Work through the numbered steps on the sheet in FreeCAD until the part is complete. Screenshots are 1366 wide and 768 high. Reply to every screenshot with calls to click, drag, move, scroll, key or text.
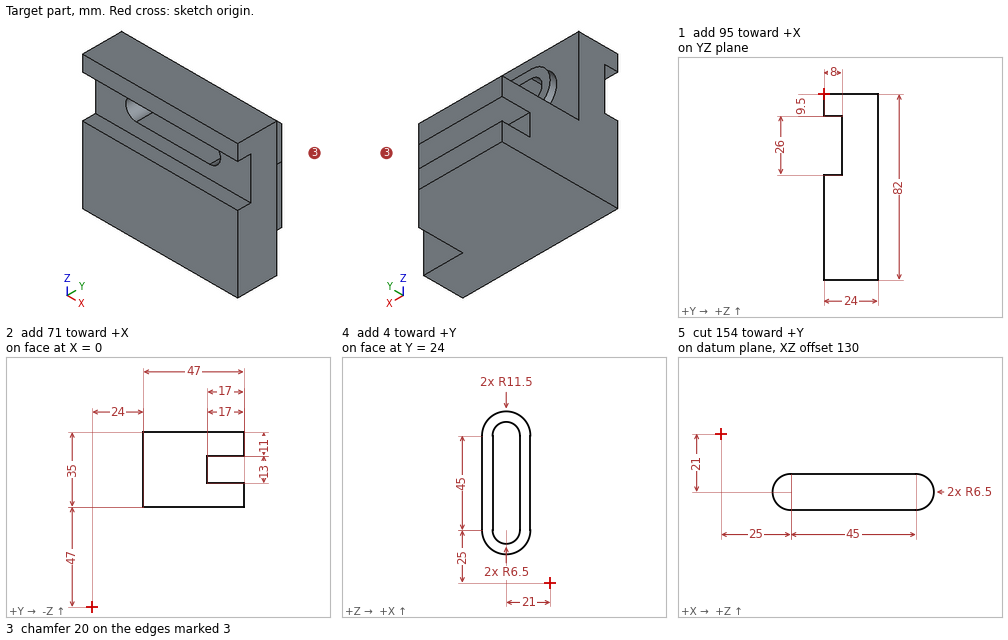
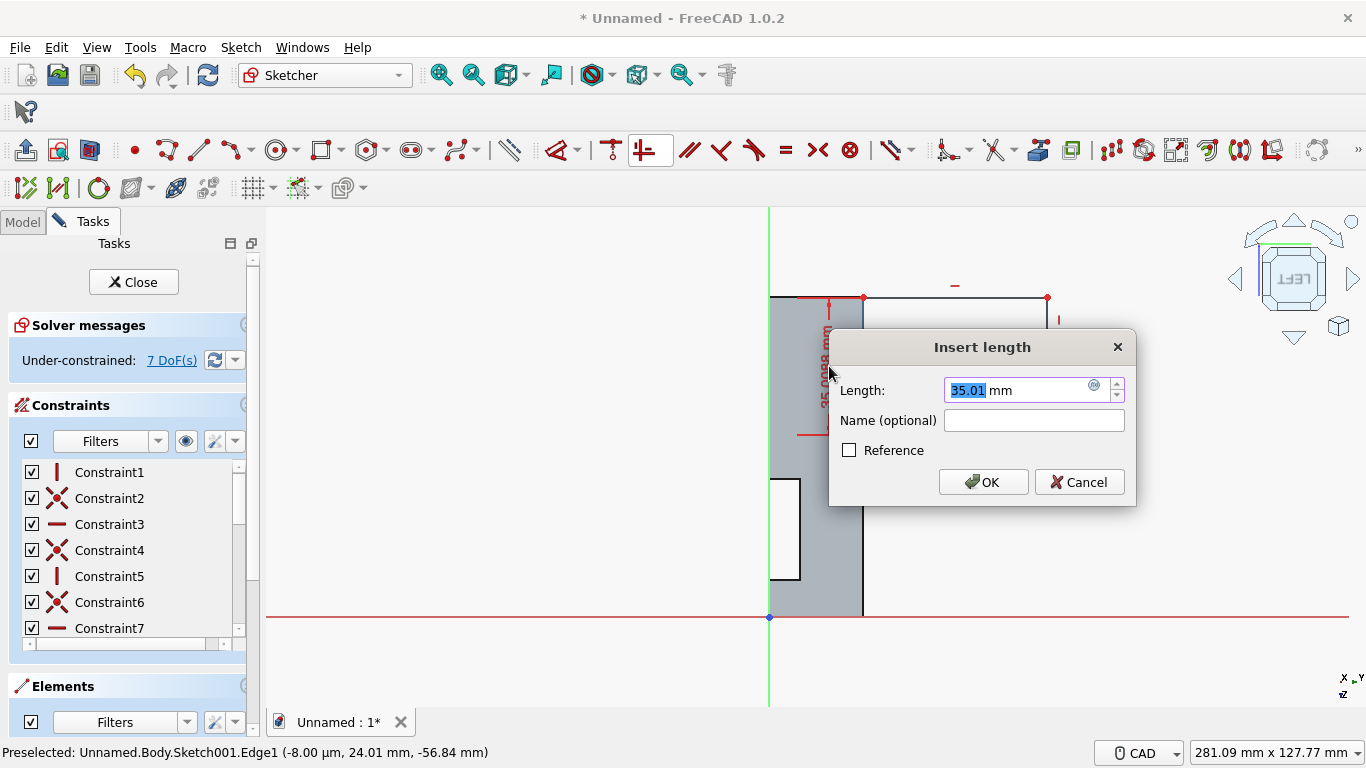
text(35)
key(Return)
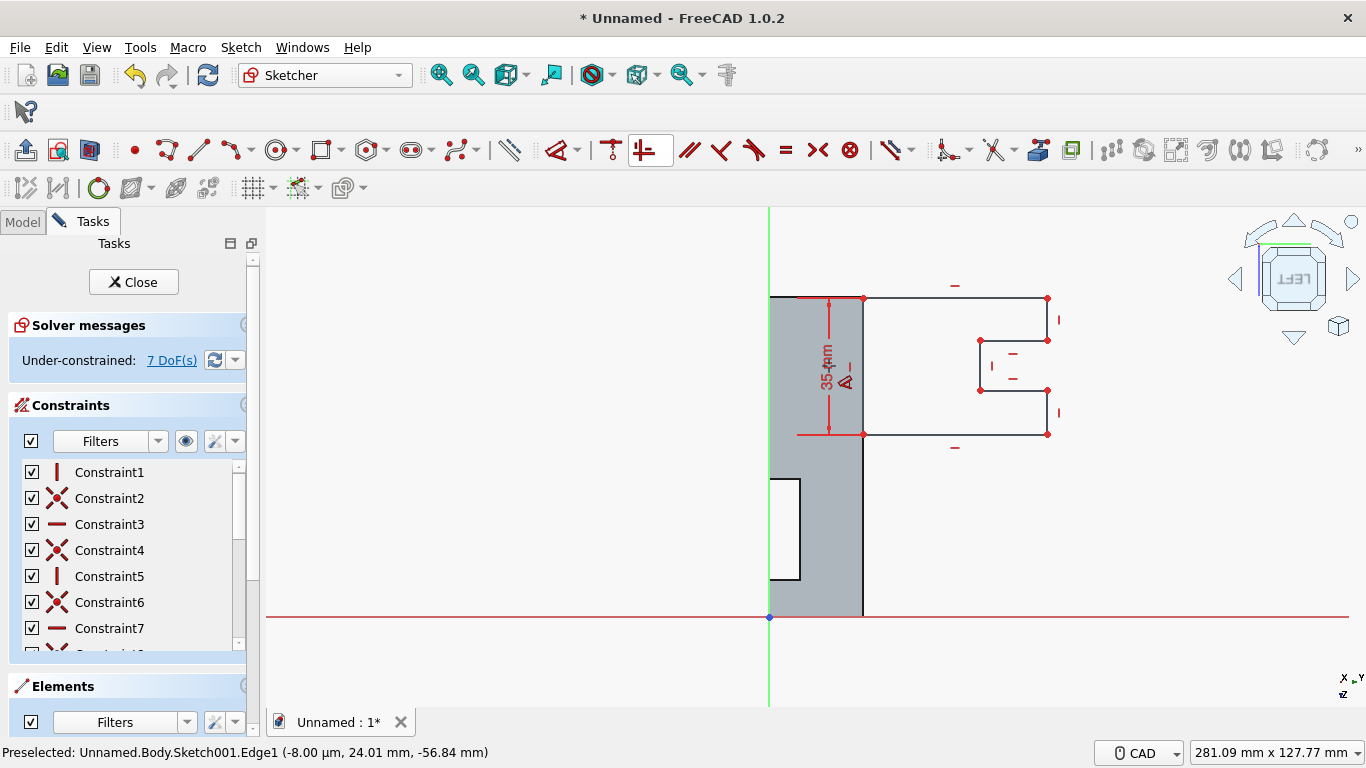
click(918, 298)
click(955, 264)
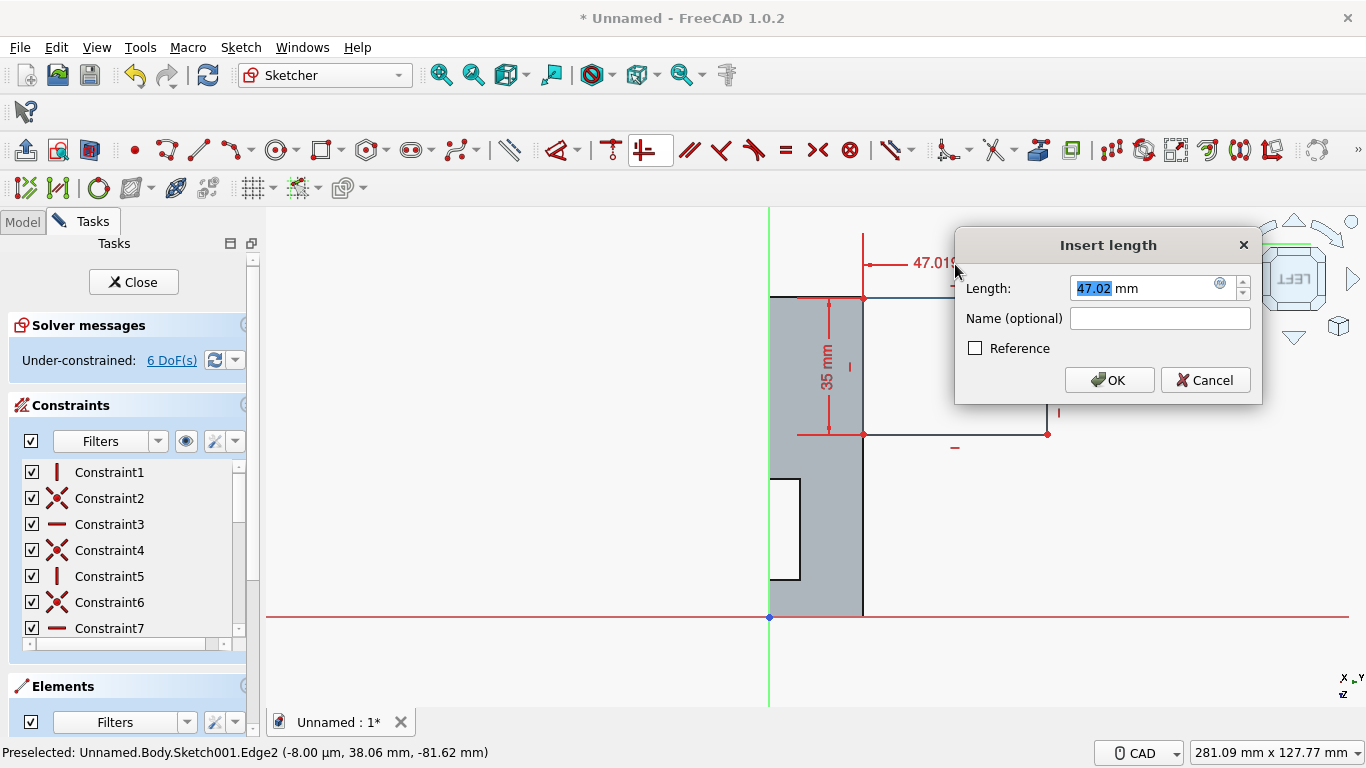
text(47)
key(Return)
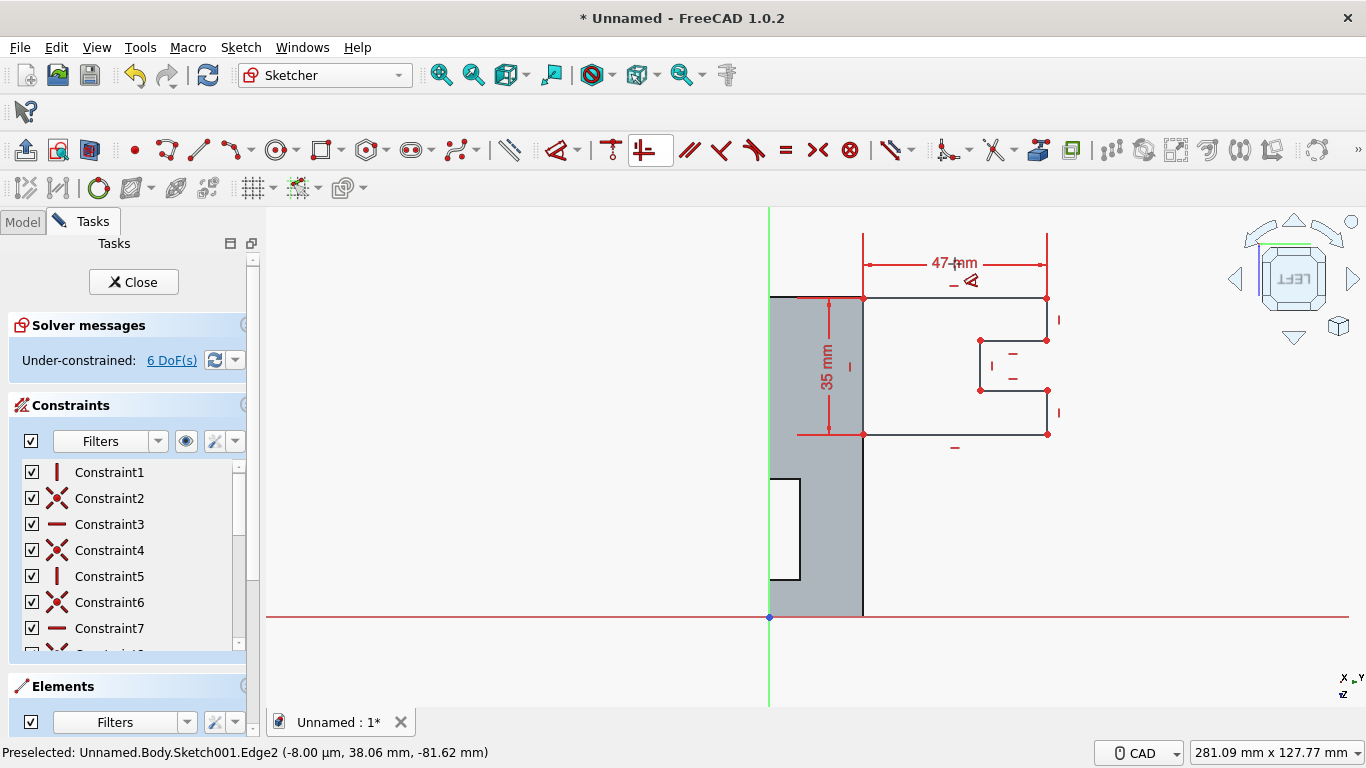
click(1047, 311)
click(1081, 320)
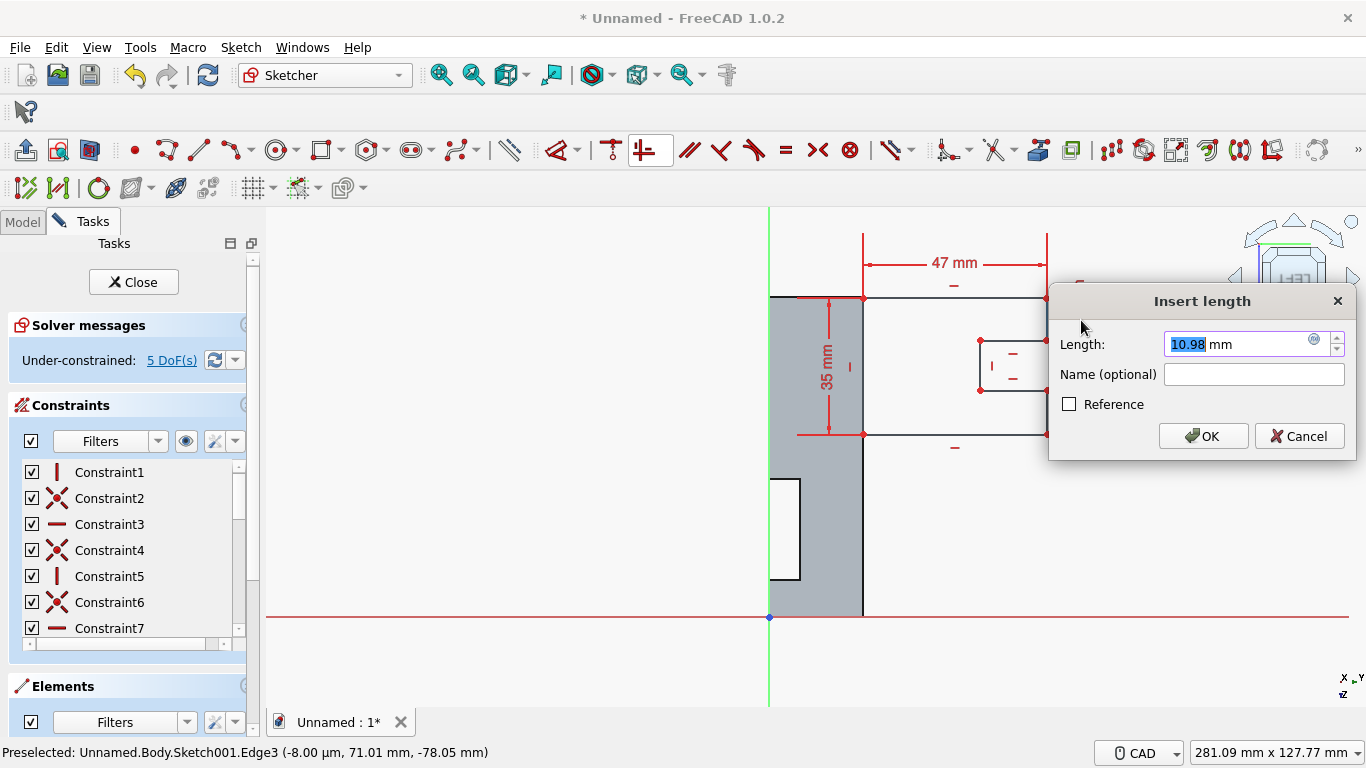
text(11)
key(Return)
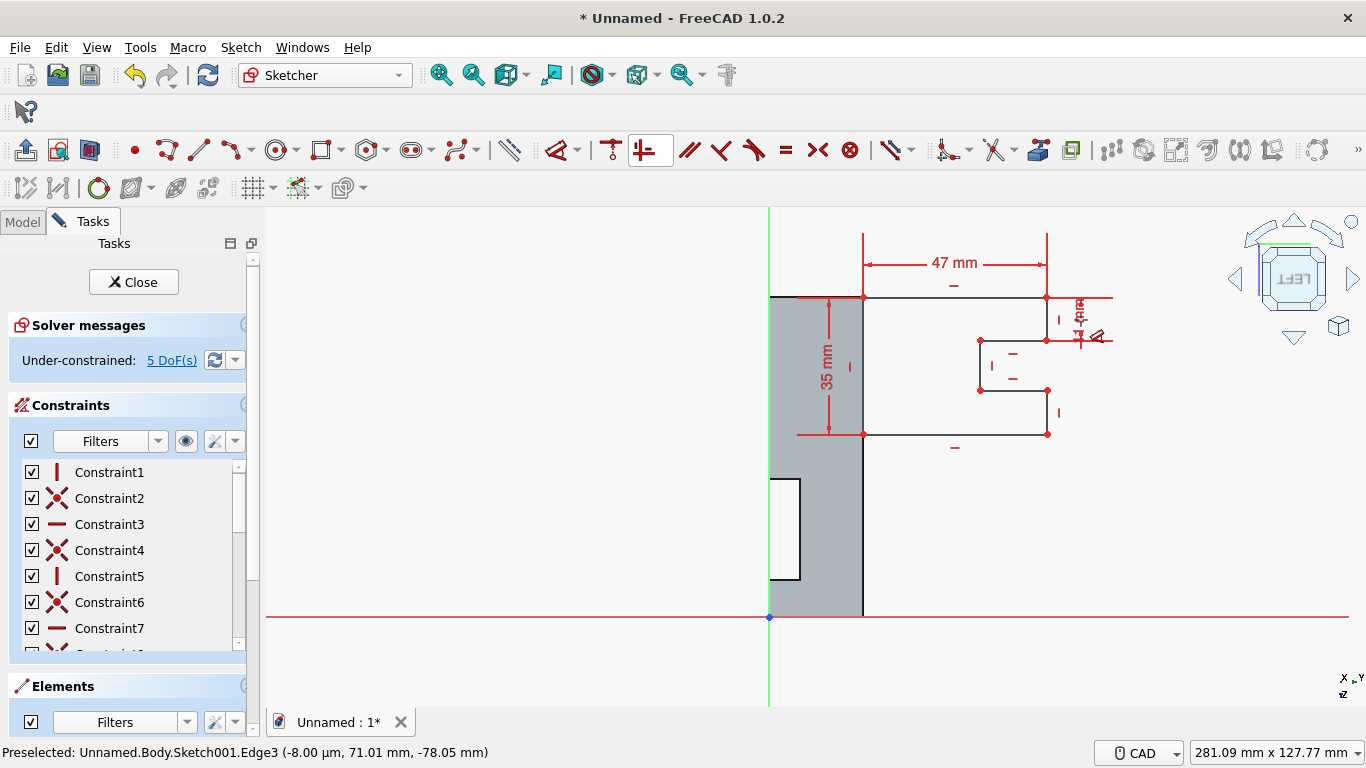
click(1027, 341)
click(1013, 375)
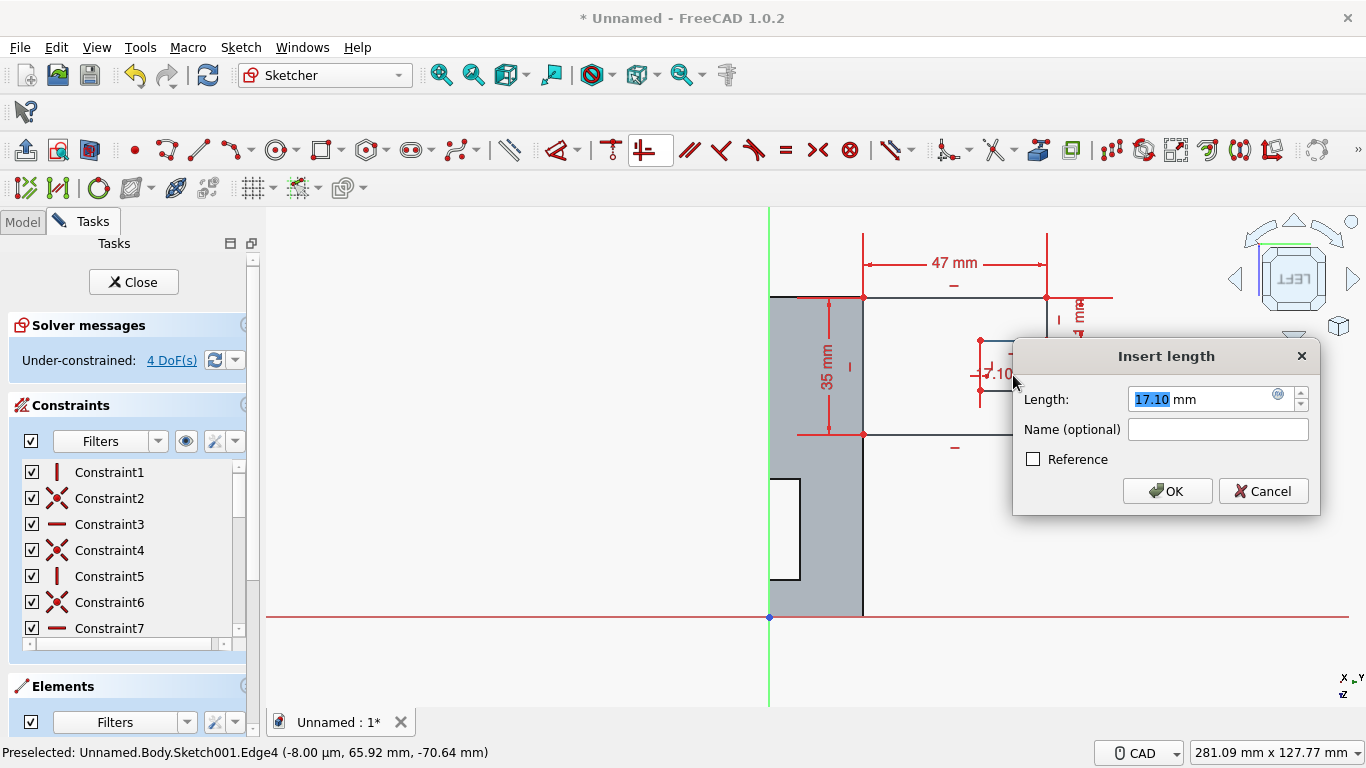
text(17)
key(Return)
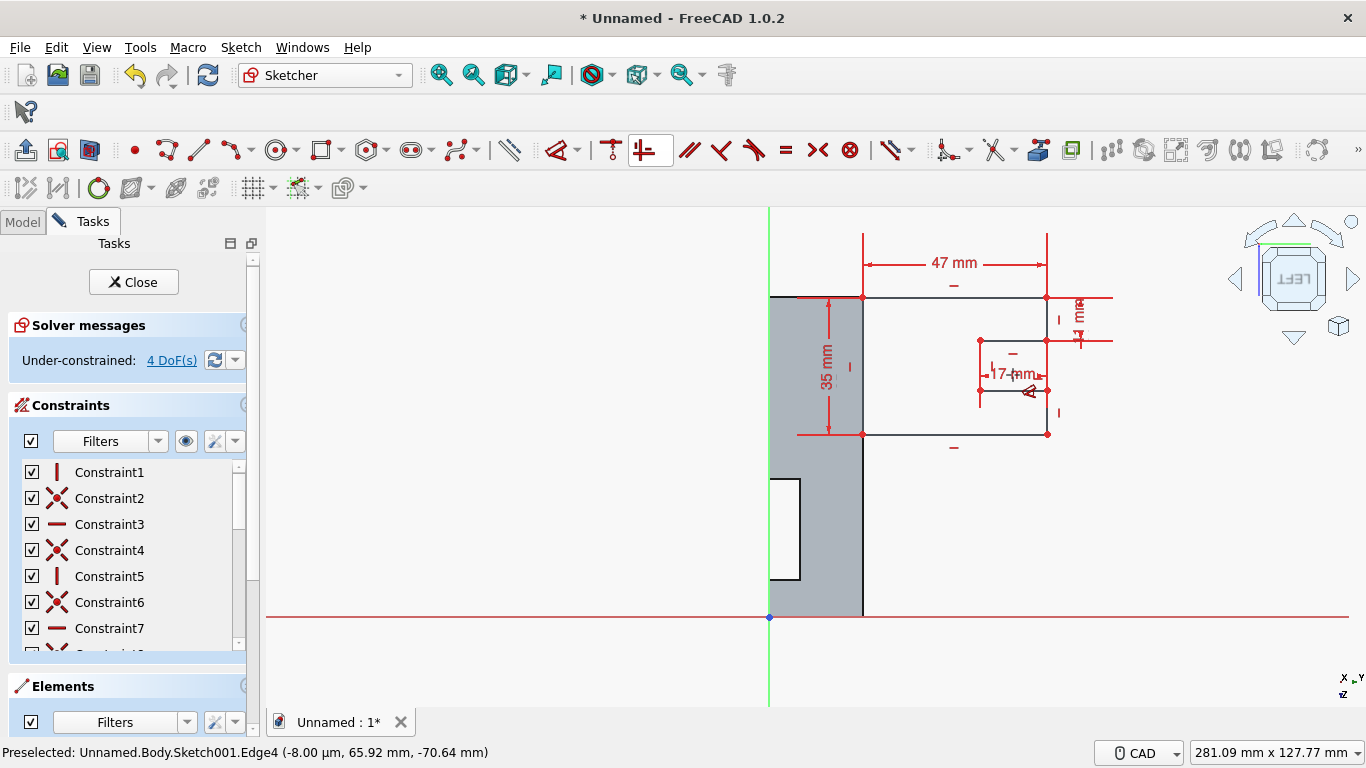
click(980, 356)
click(1014, 355)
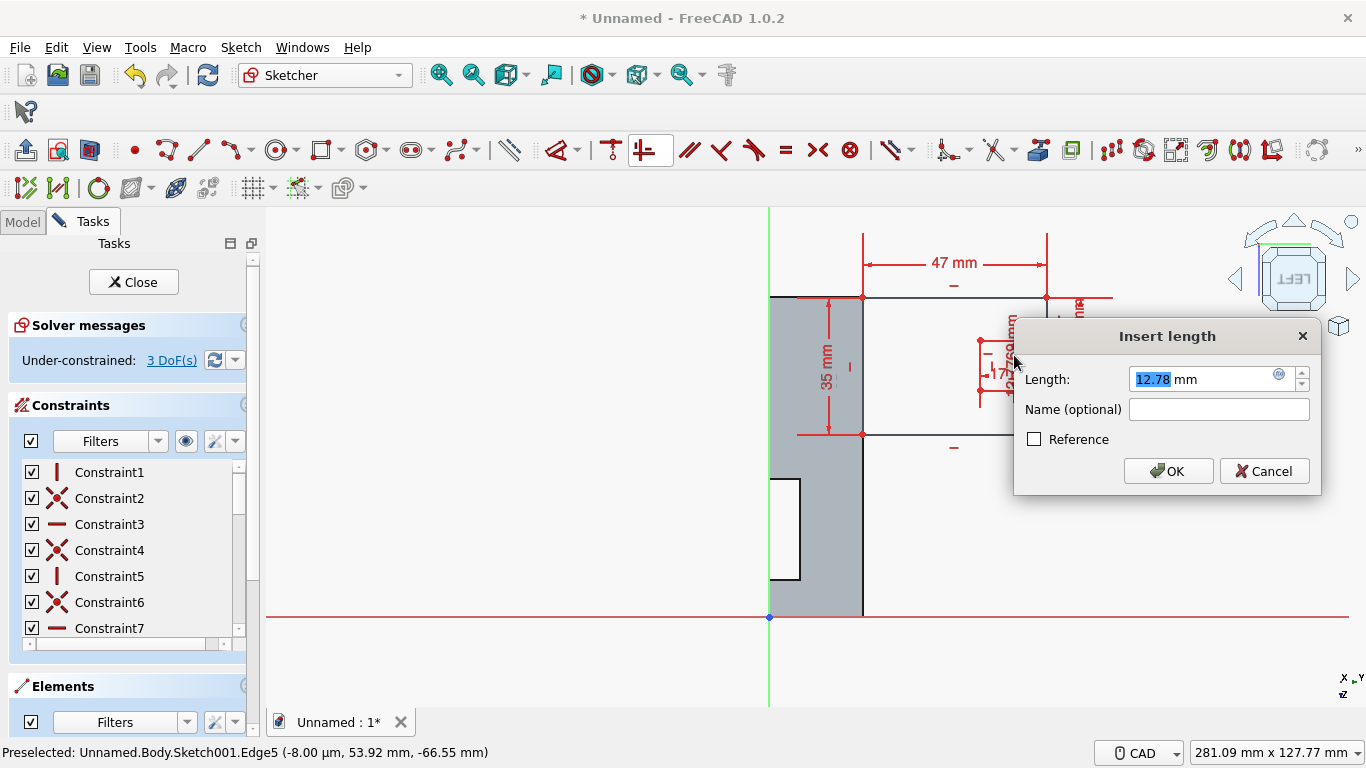
text(13)
key(Return)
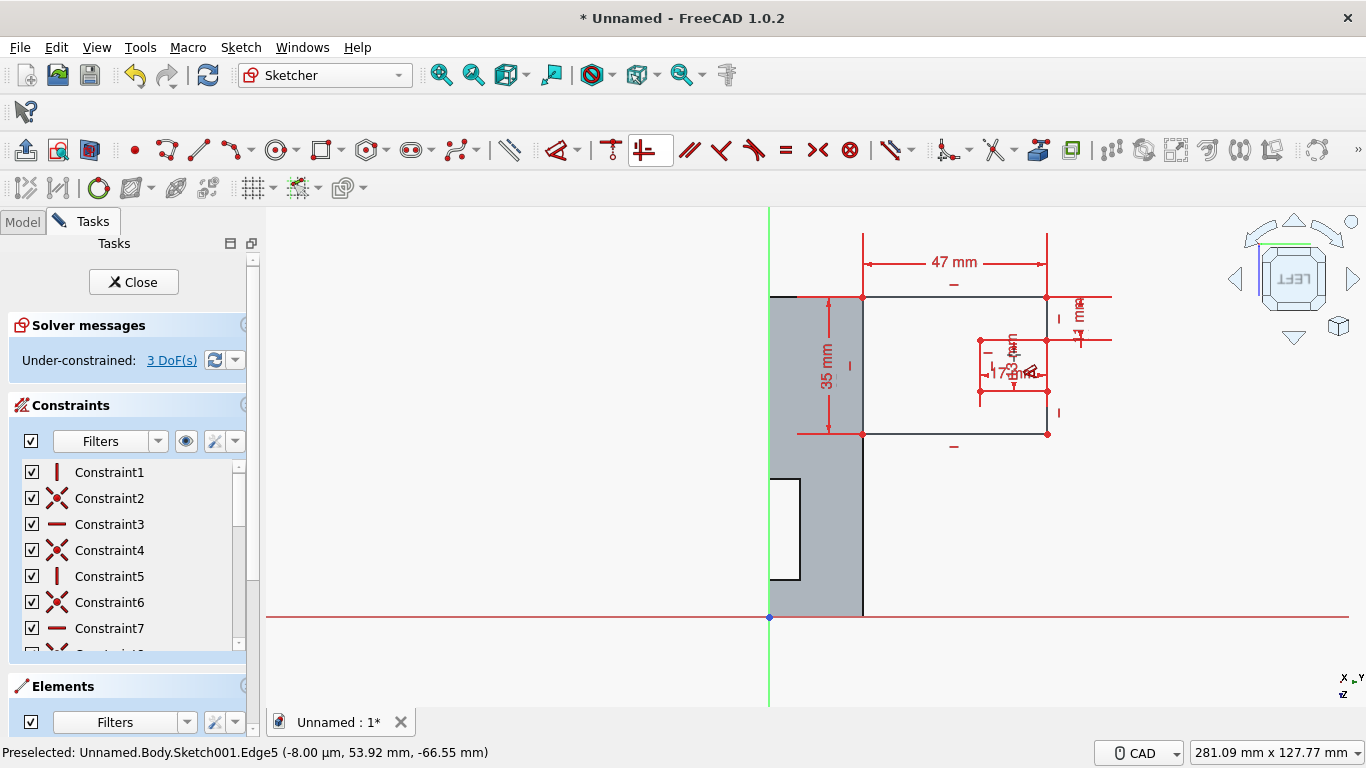
click(1000, 391)
click(1014, 449)